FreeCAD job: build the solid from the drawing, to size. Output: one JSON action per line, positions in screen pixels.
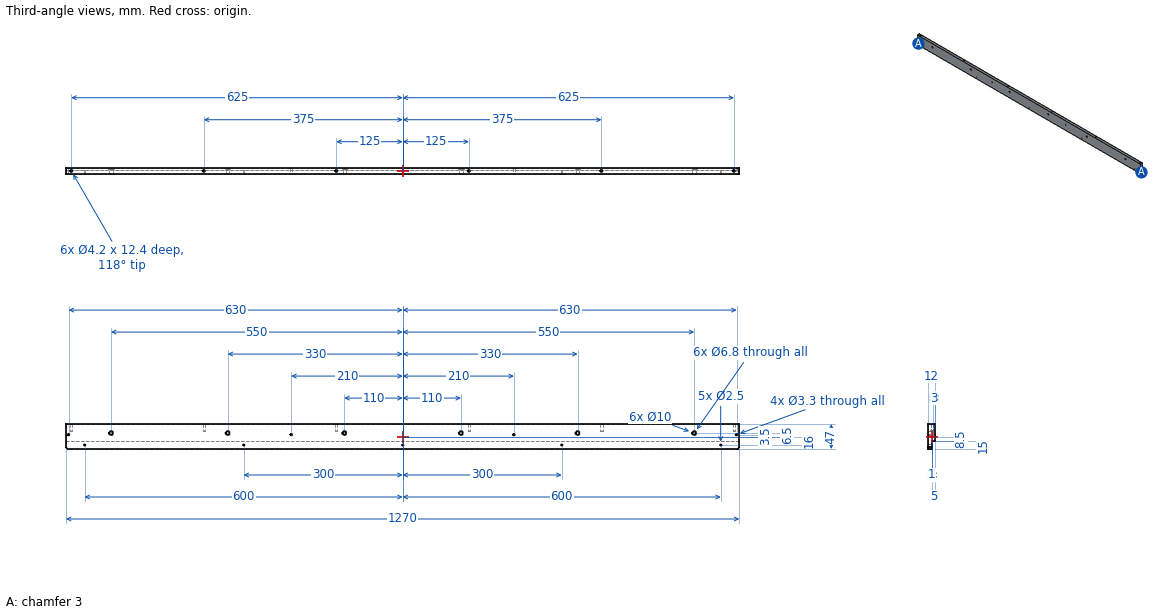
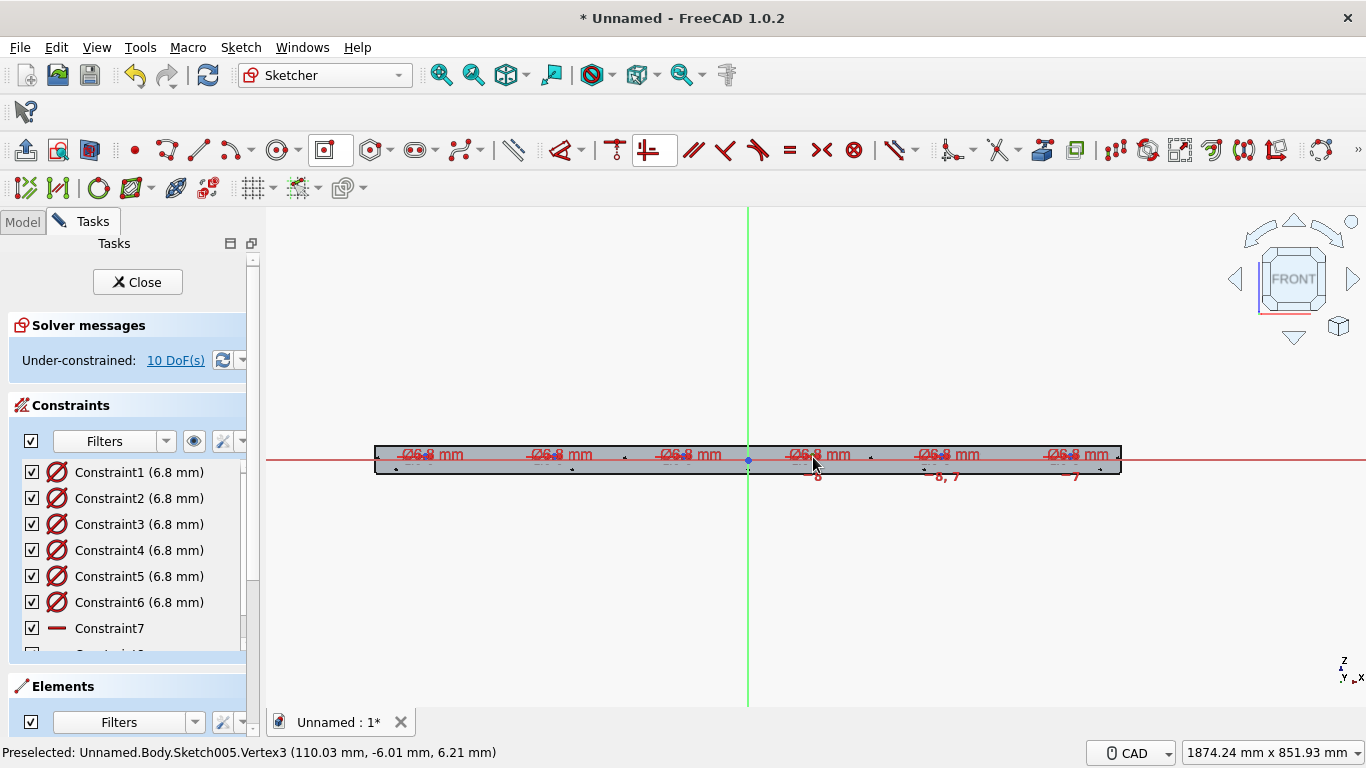
{"action": "left_click", "coordinate": [684, 457]}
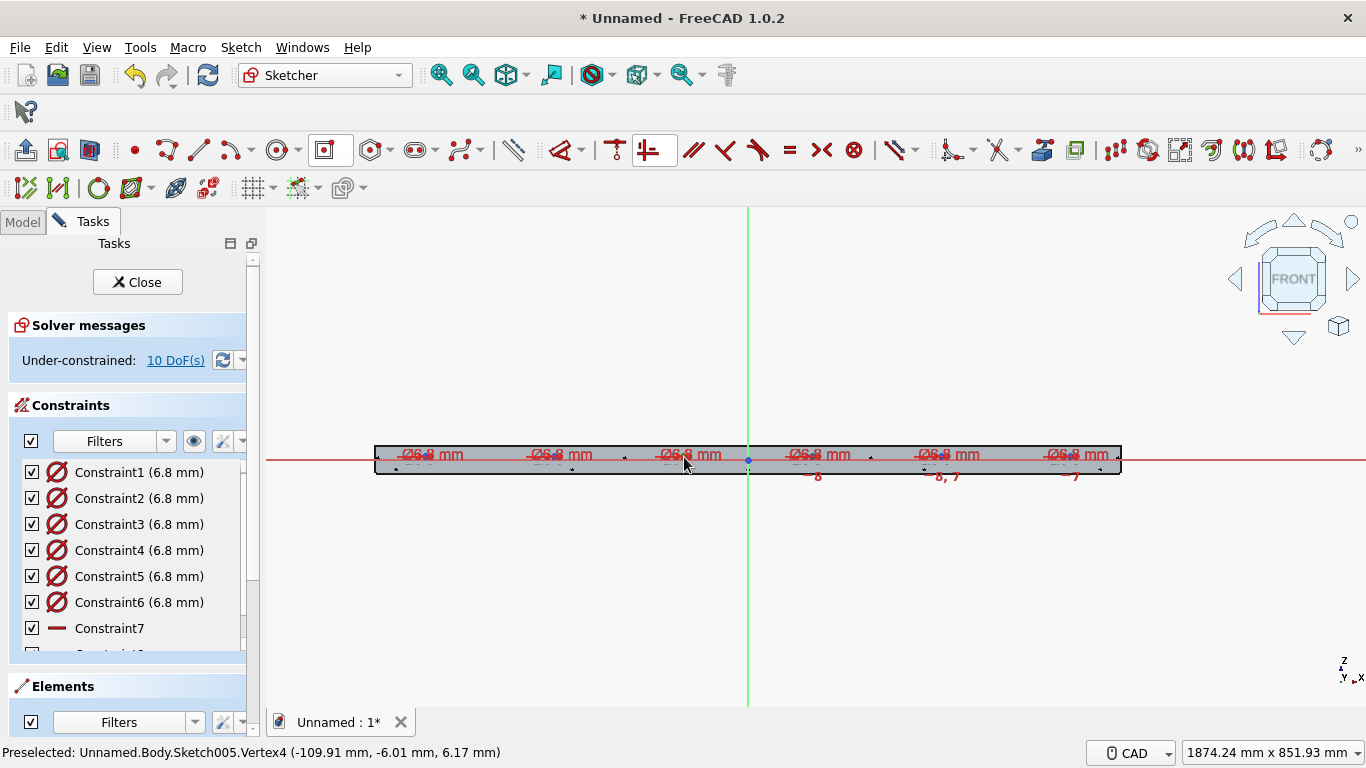
{"action": "left_click", "coordinate": [672, 150]}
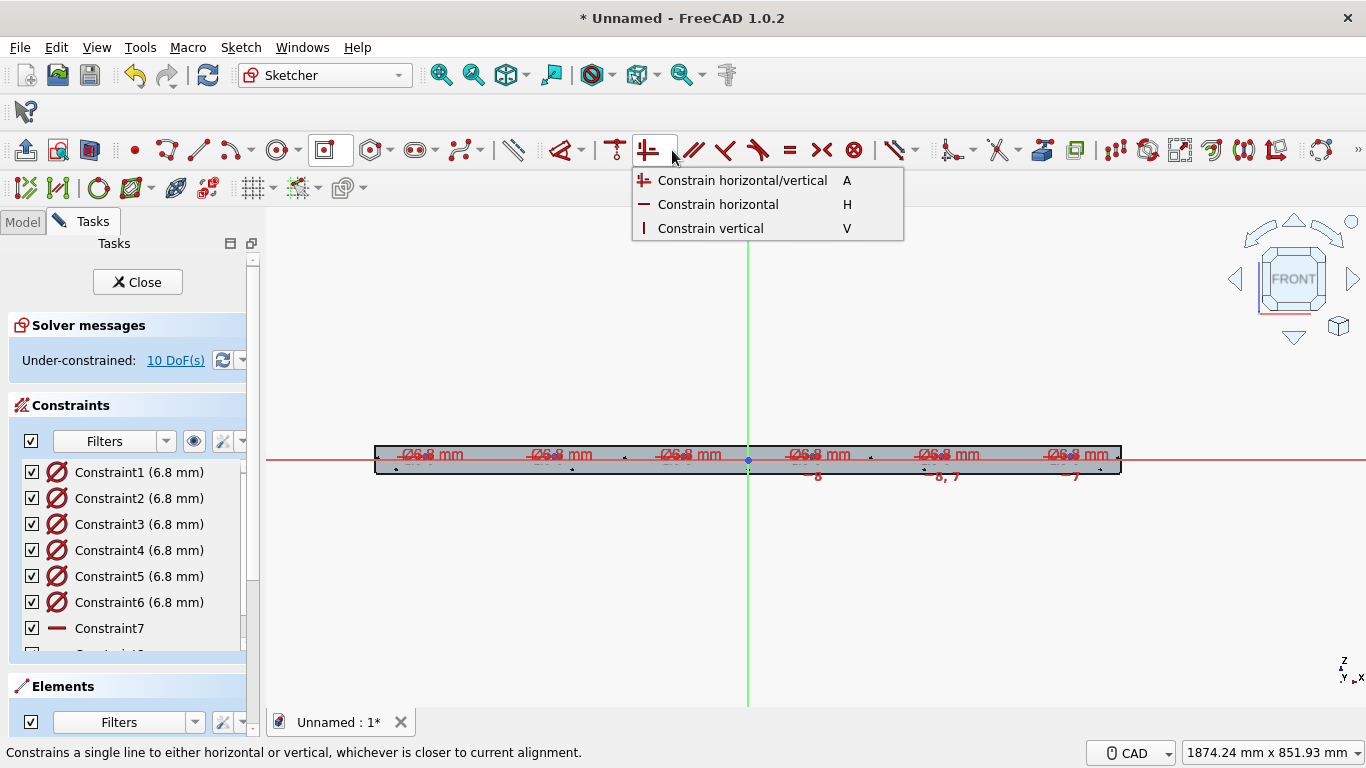
{"action": "left_click", "coordinate": [768, 204]}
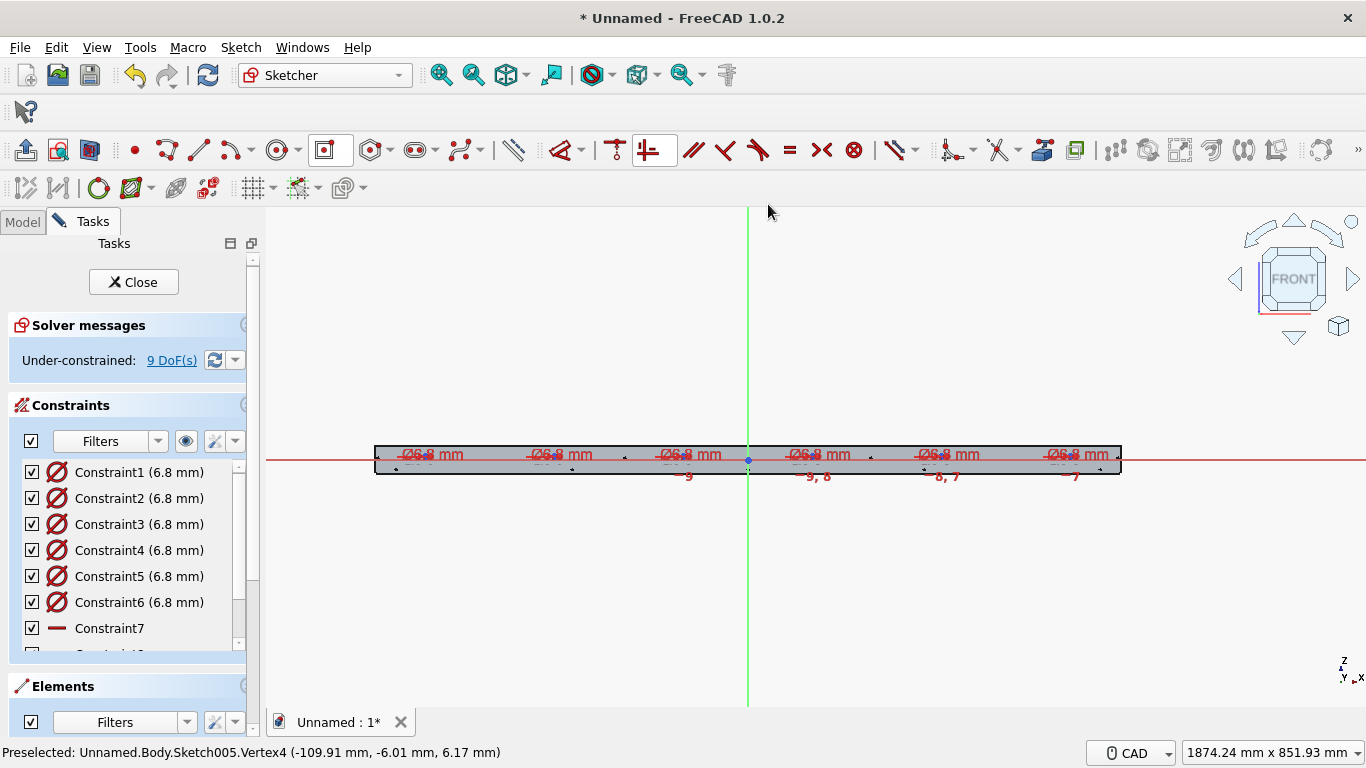
{"action": "left_click", "coordinate": [684, 457]}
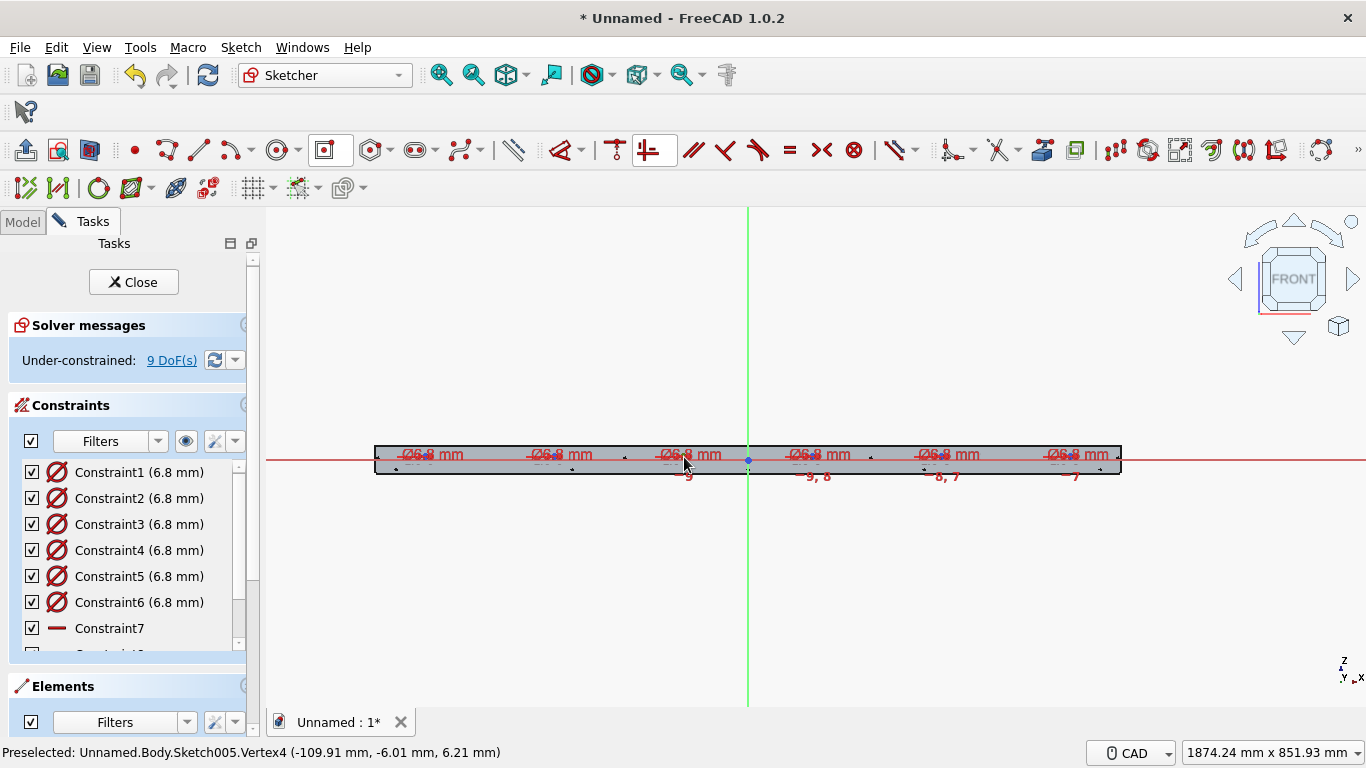
{"action": "left_click", "coordinate": [554, 457]}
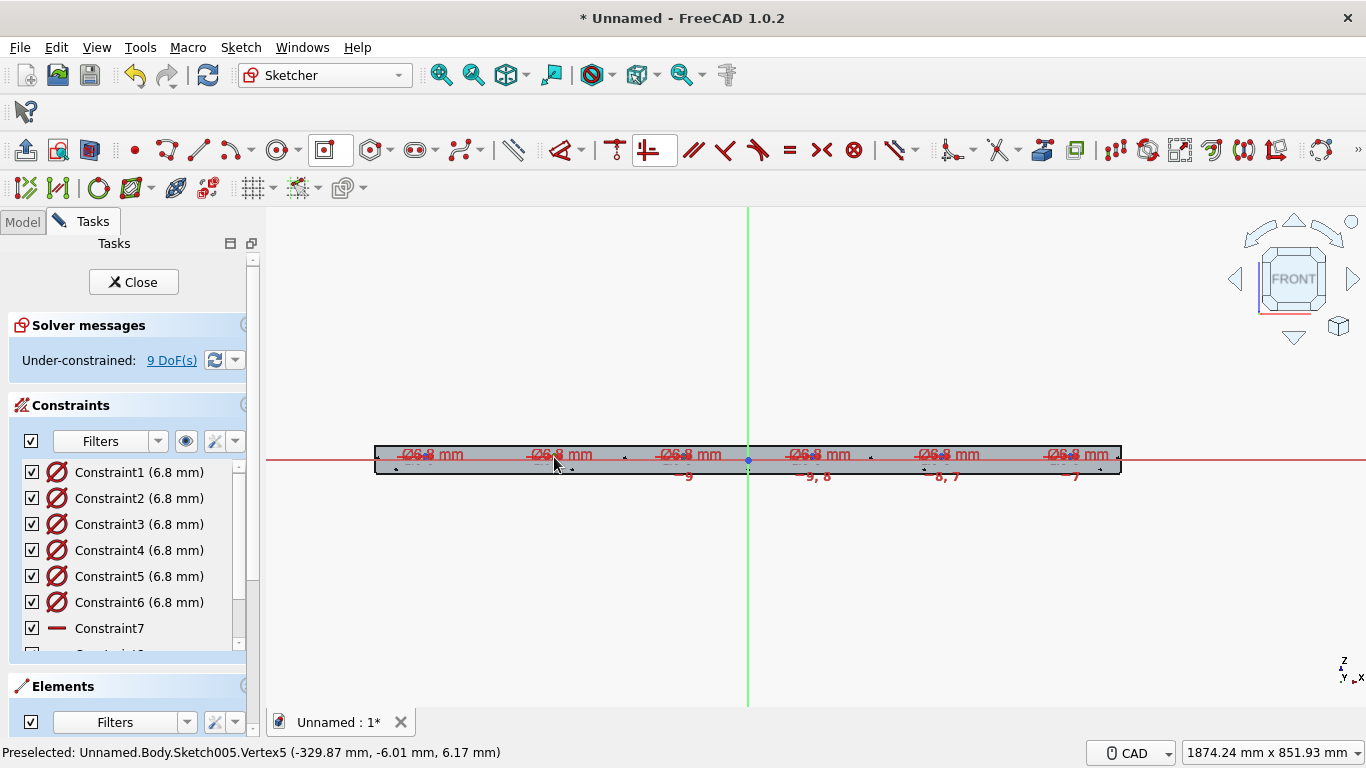
{"action": "left_click", "coordinate": [672, 150]}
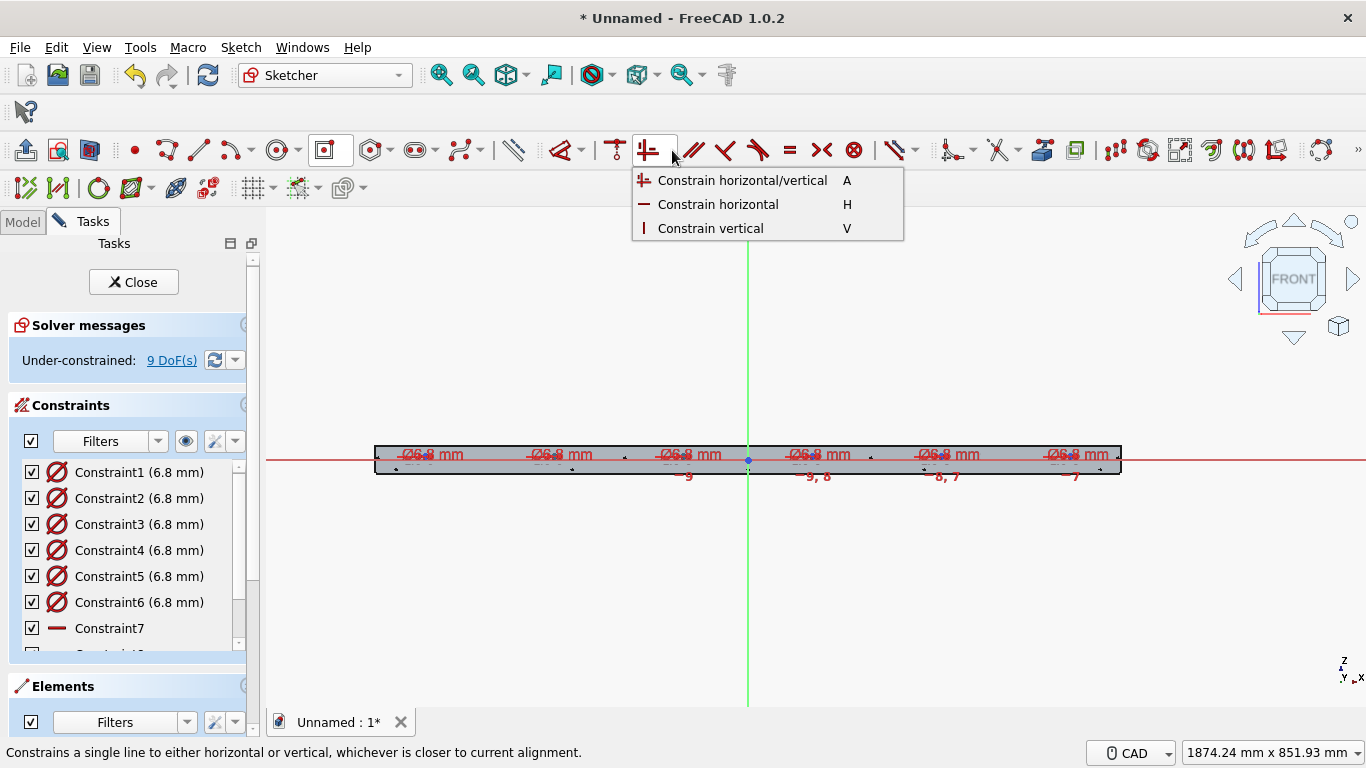
{"action": "left_click", "coordinate": [768, 204]}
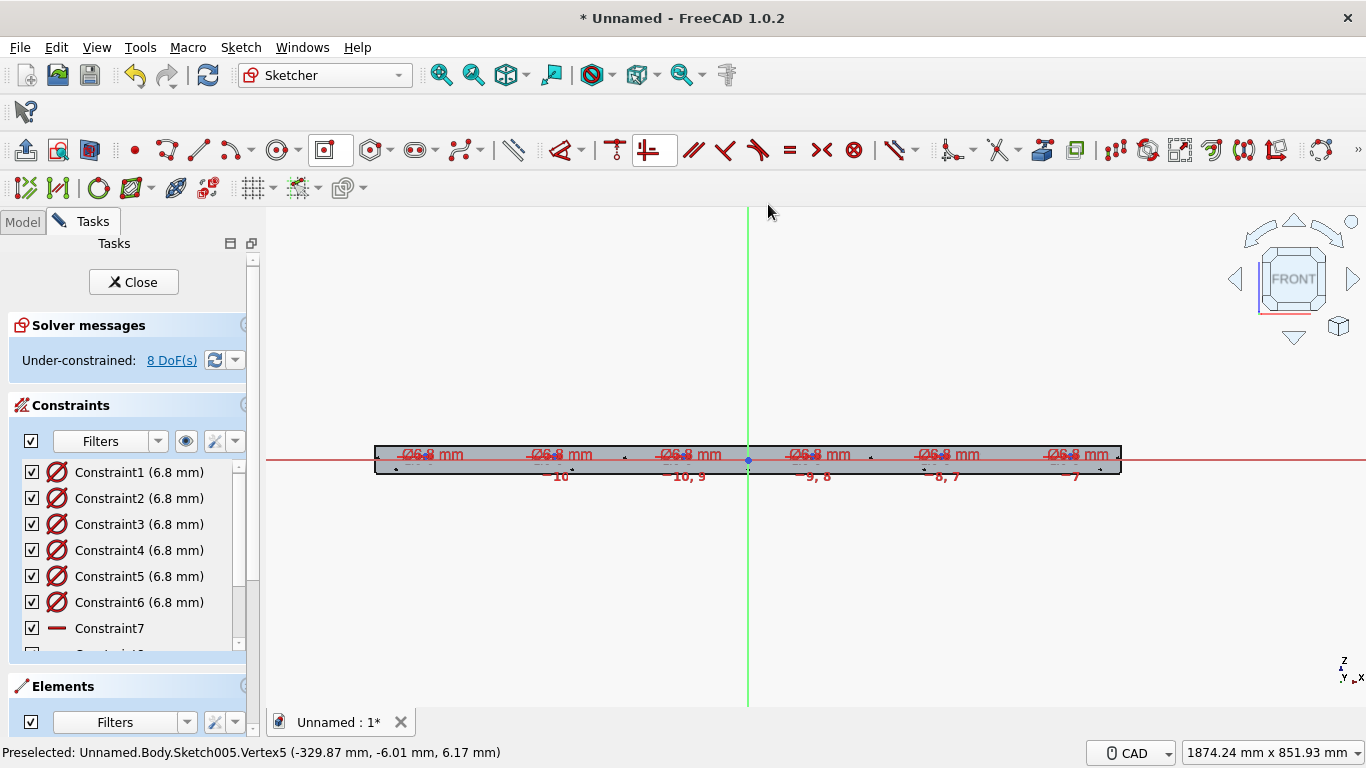
{"action": "left_click", "coordinate": [554, 457]}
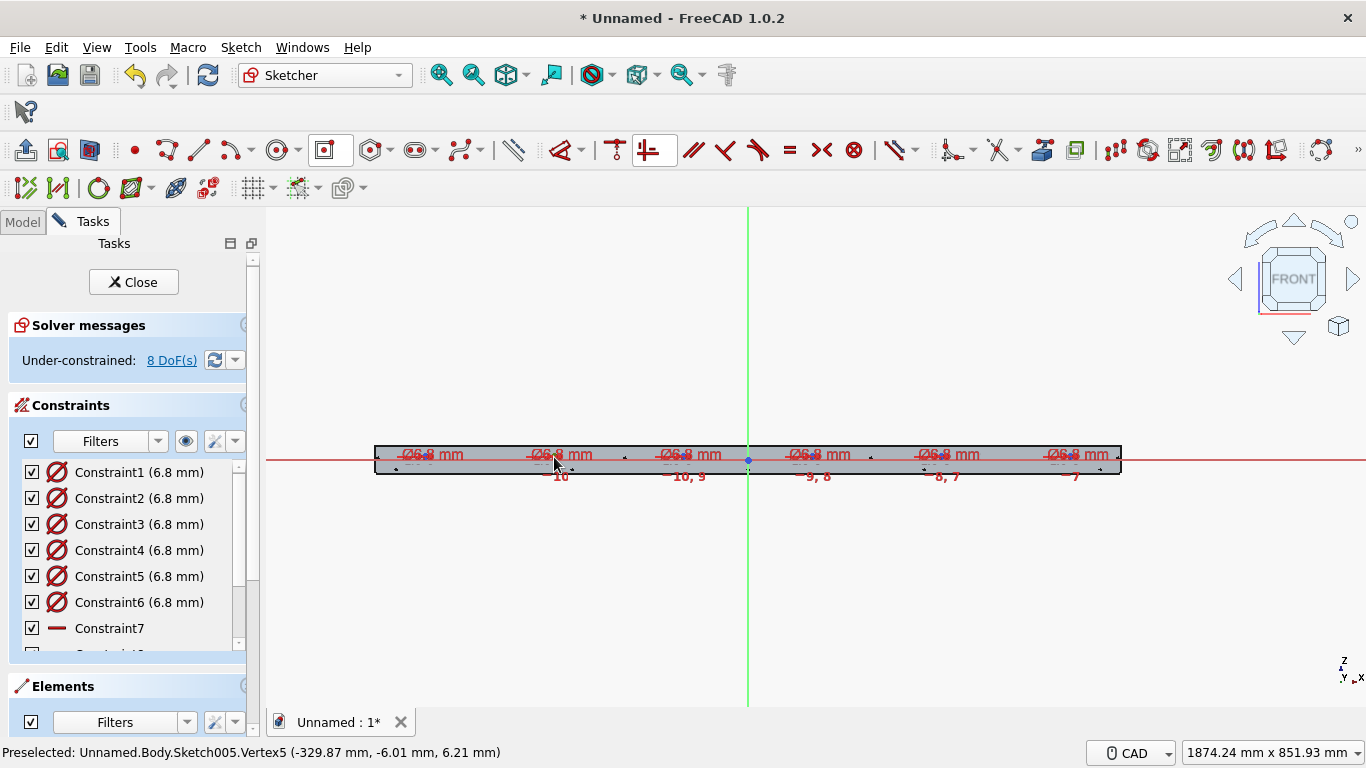
{"action": "left_click", "coordinate": [425, 457]}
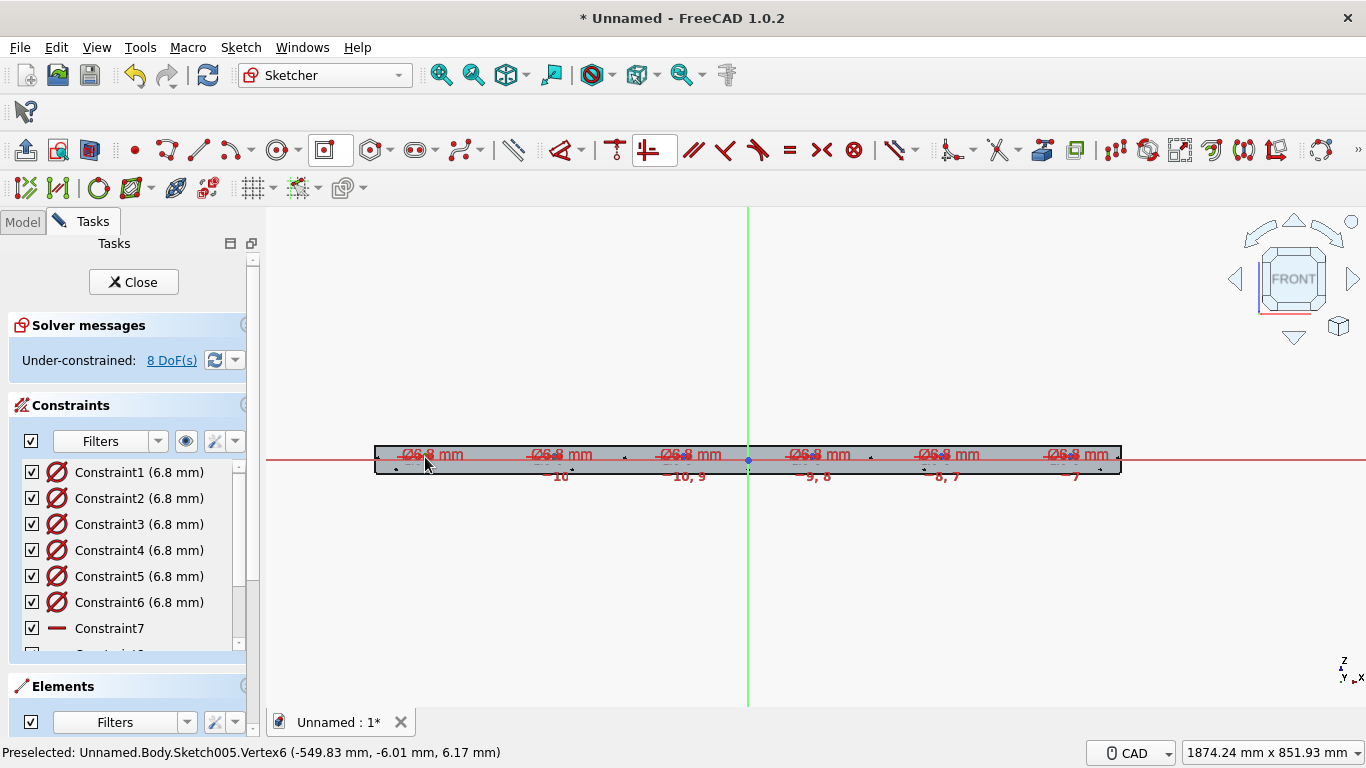
{"action": "key", "text": "h"}